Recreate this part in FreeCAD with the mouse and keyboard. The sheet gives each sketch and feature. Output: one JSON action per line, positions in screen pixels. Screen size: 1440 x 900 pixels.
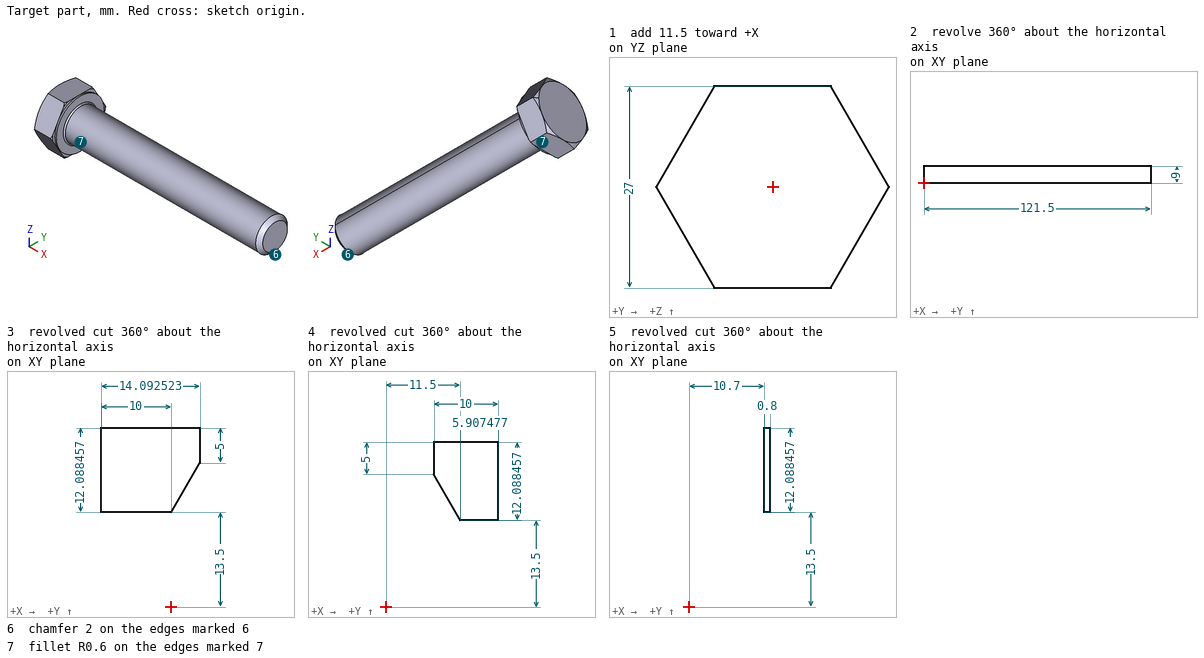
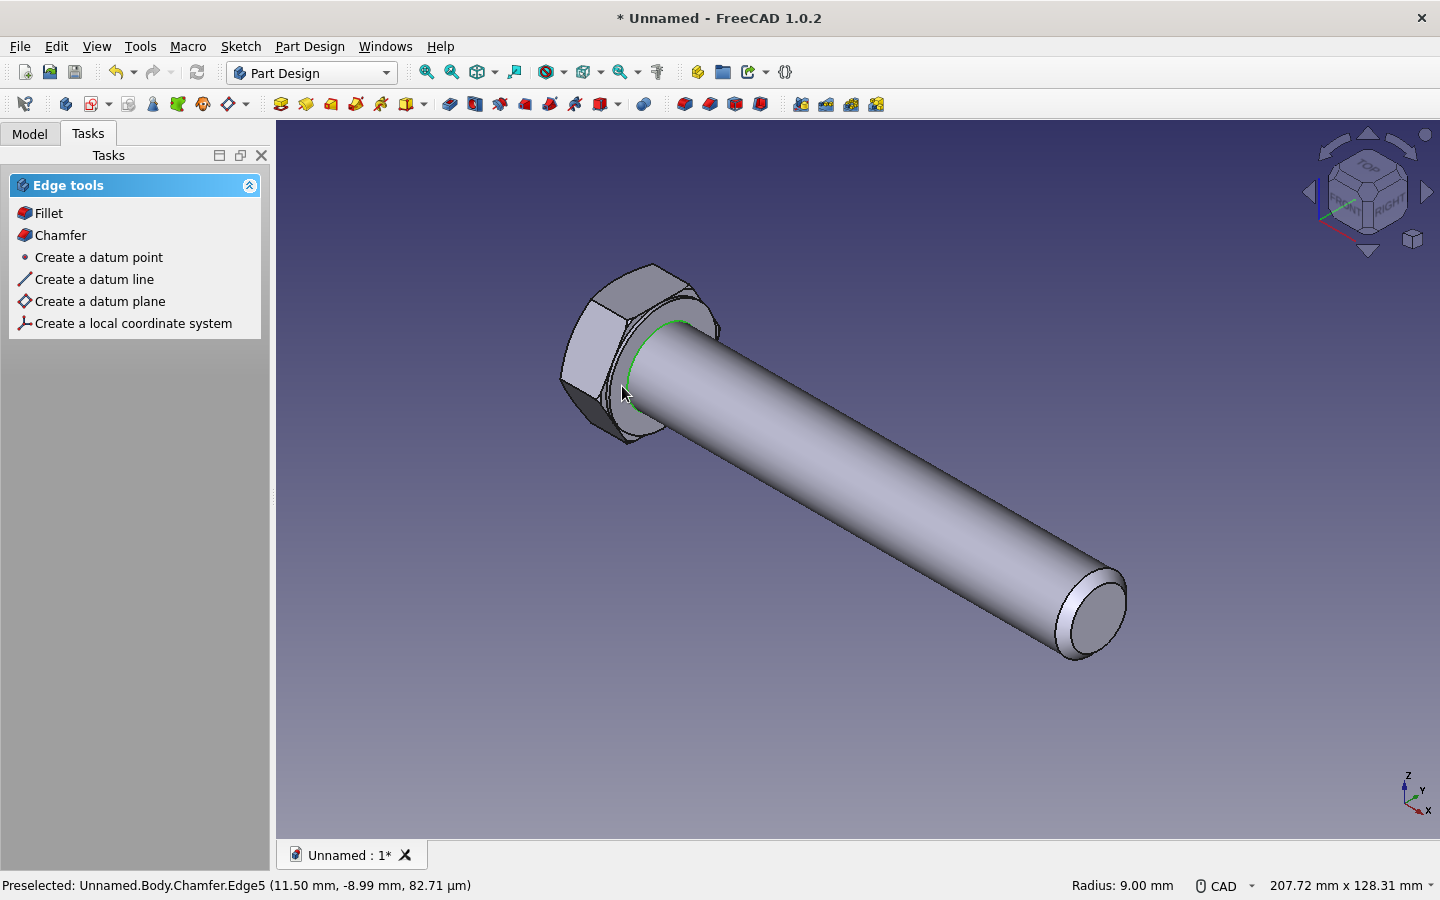
{"action": "left_click", "coordinate": [685, 104]}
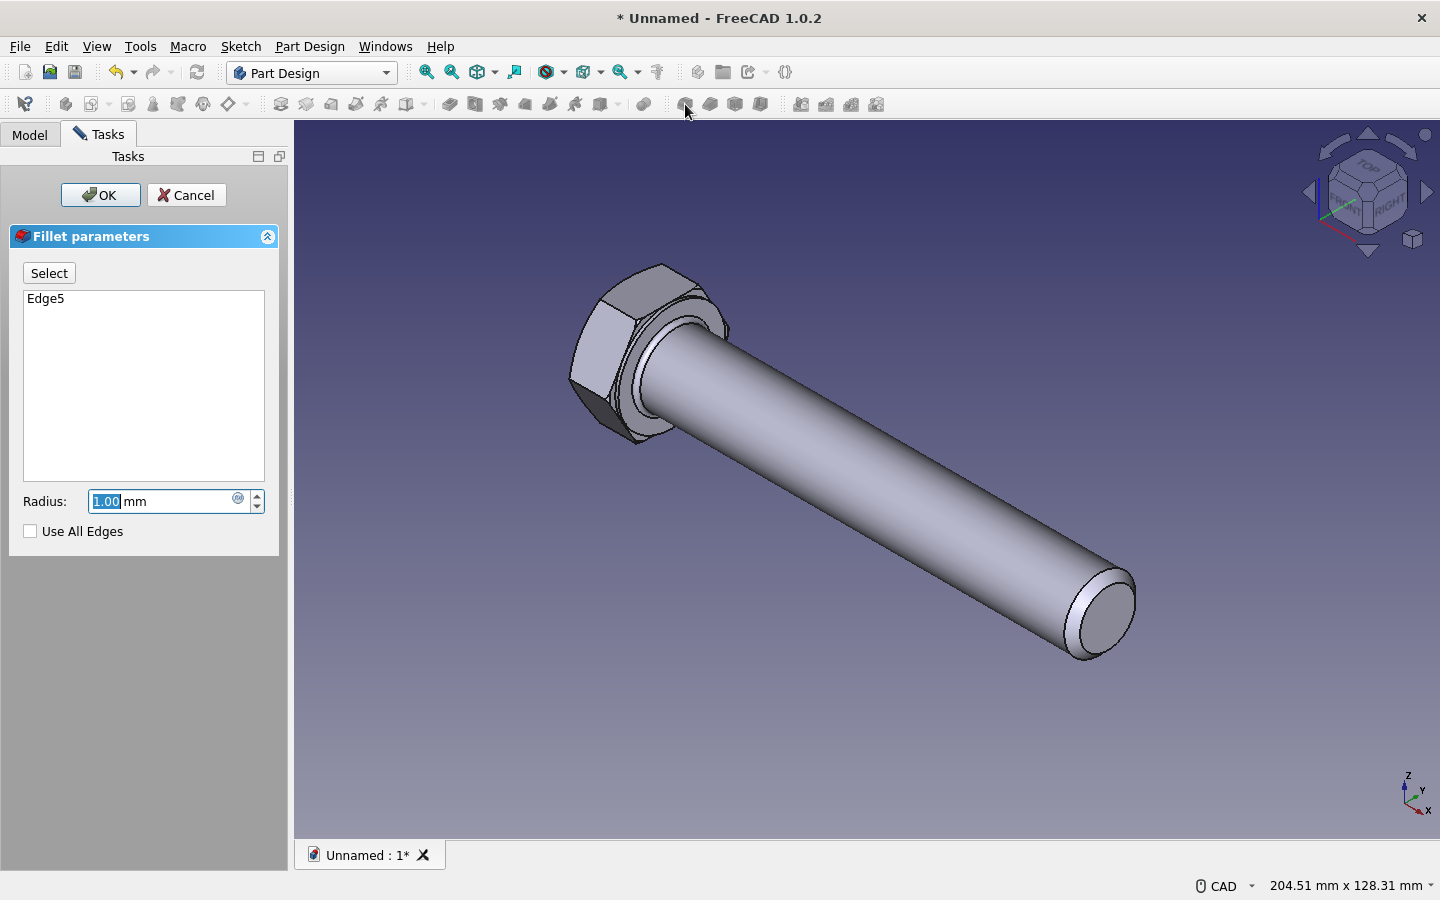
{"action": "type", "text": "0.6"}
{"action": "key", "text": "Tab"}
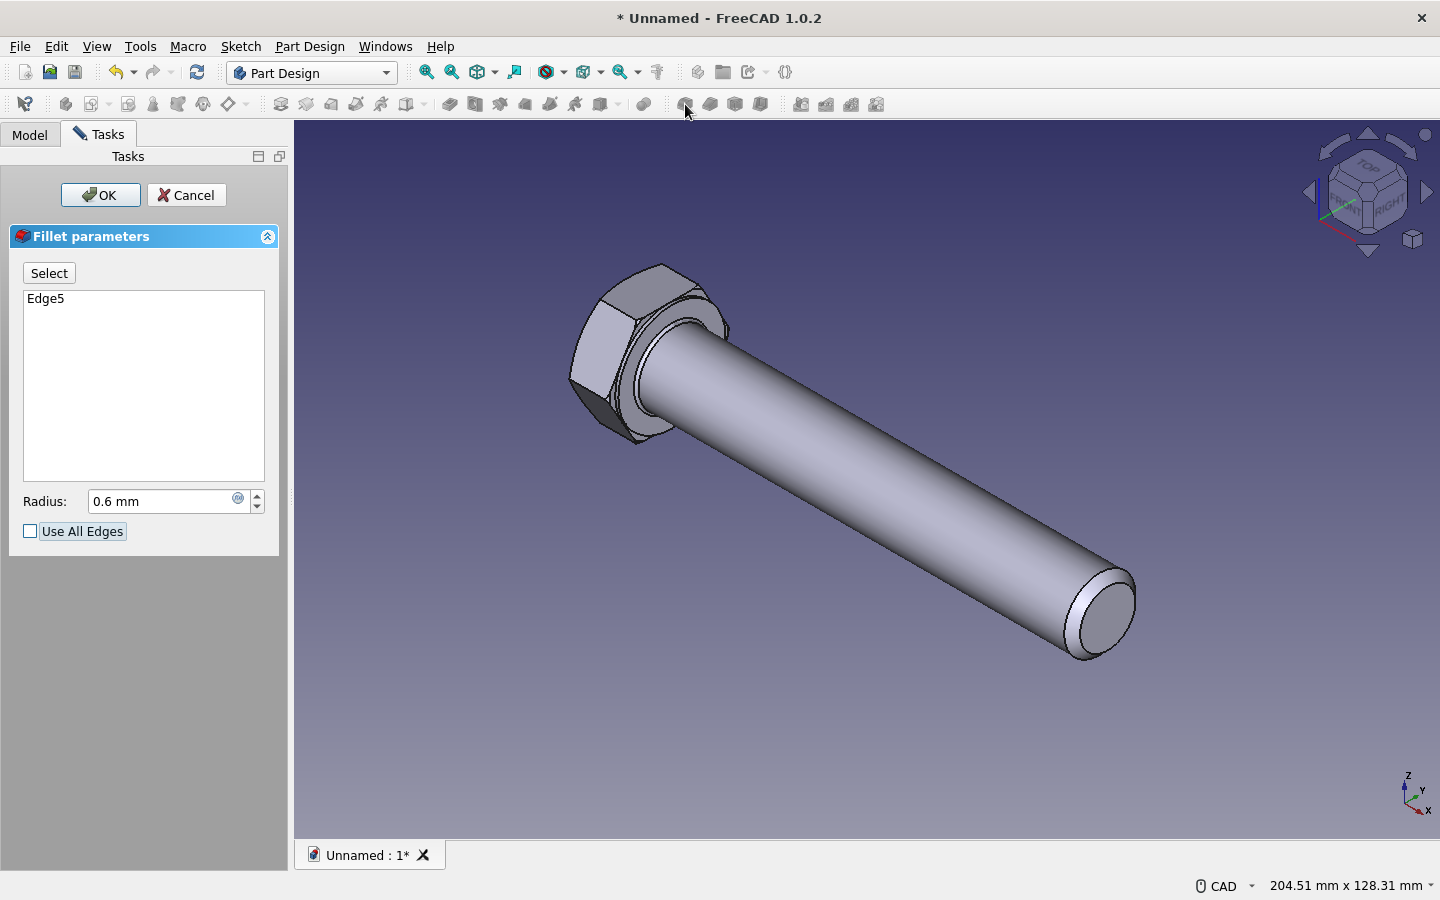
{"action": "left_click", "coordinate": [101, 195]}